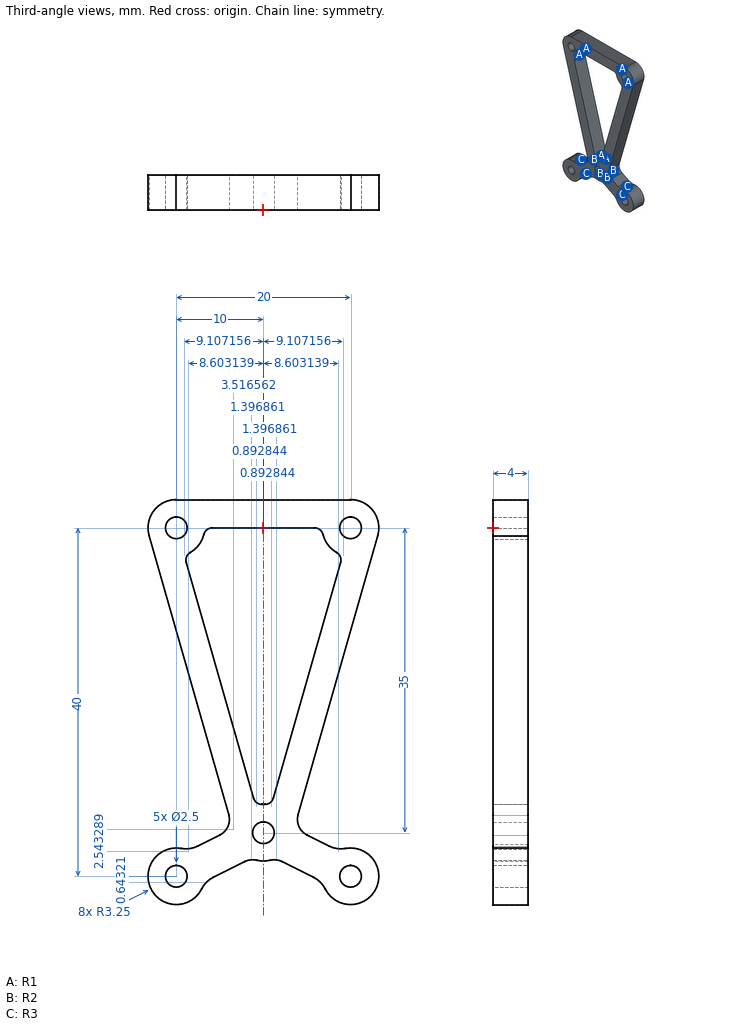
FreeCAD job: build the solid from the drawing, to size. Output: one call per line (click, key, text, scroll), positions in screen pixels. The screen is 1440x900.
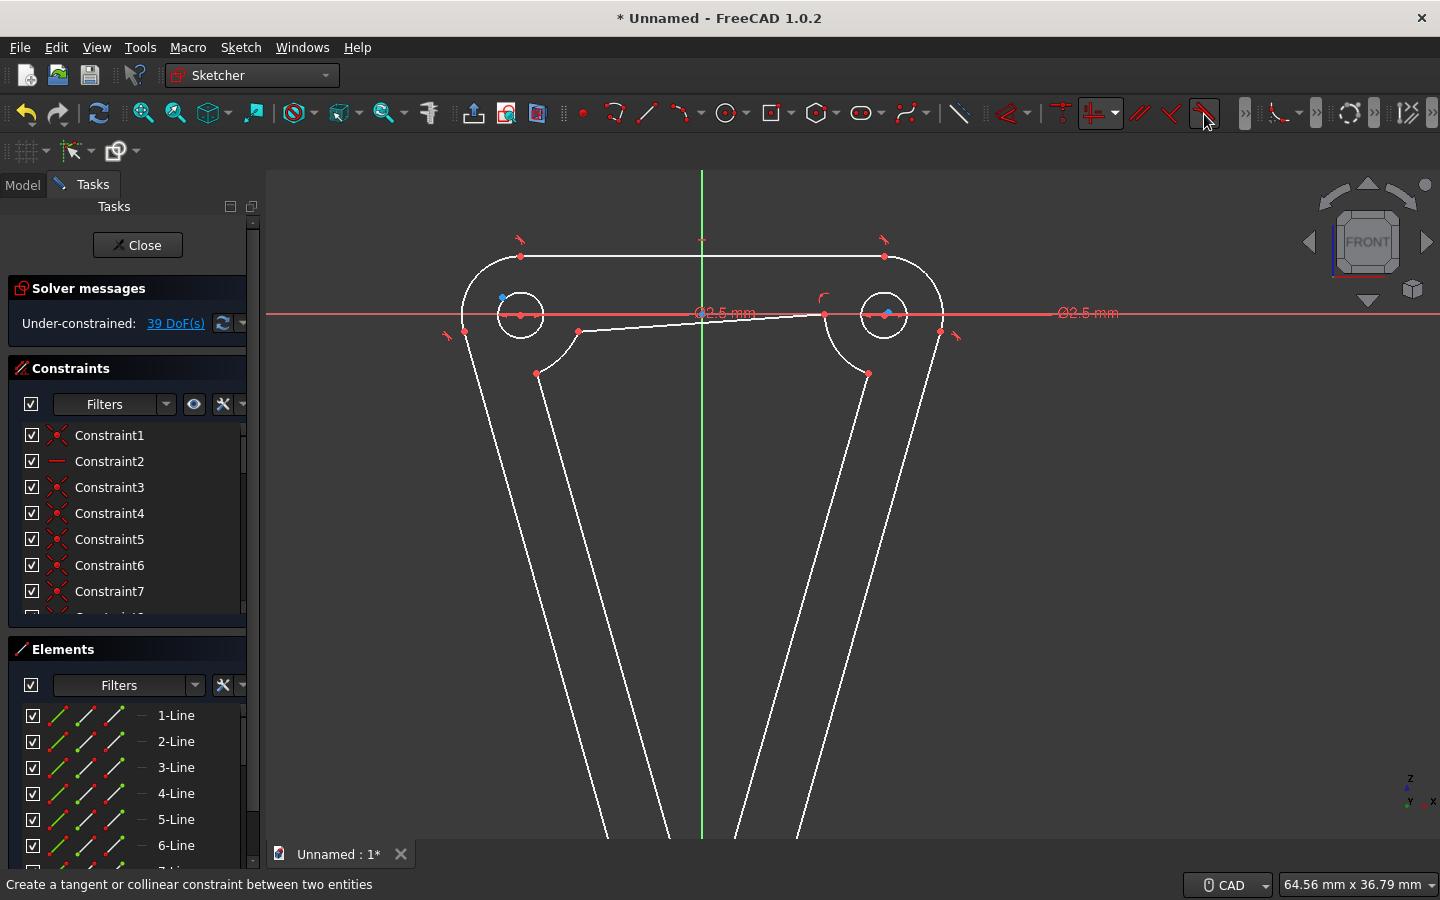
click(653, 327)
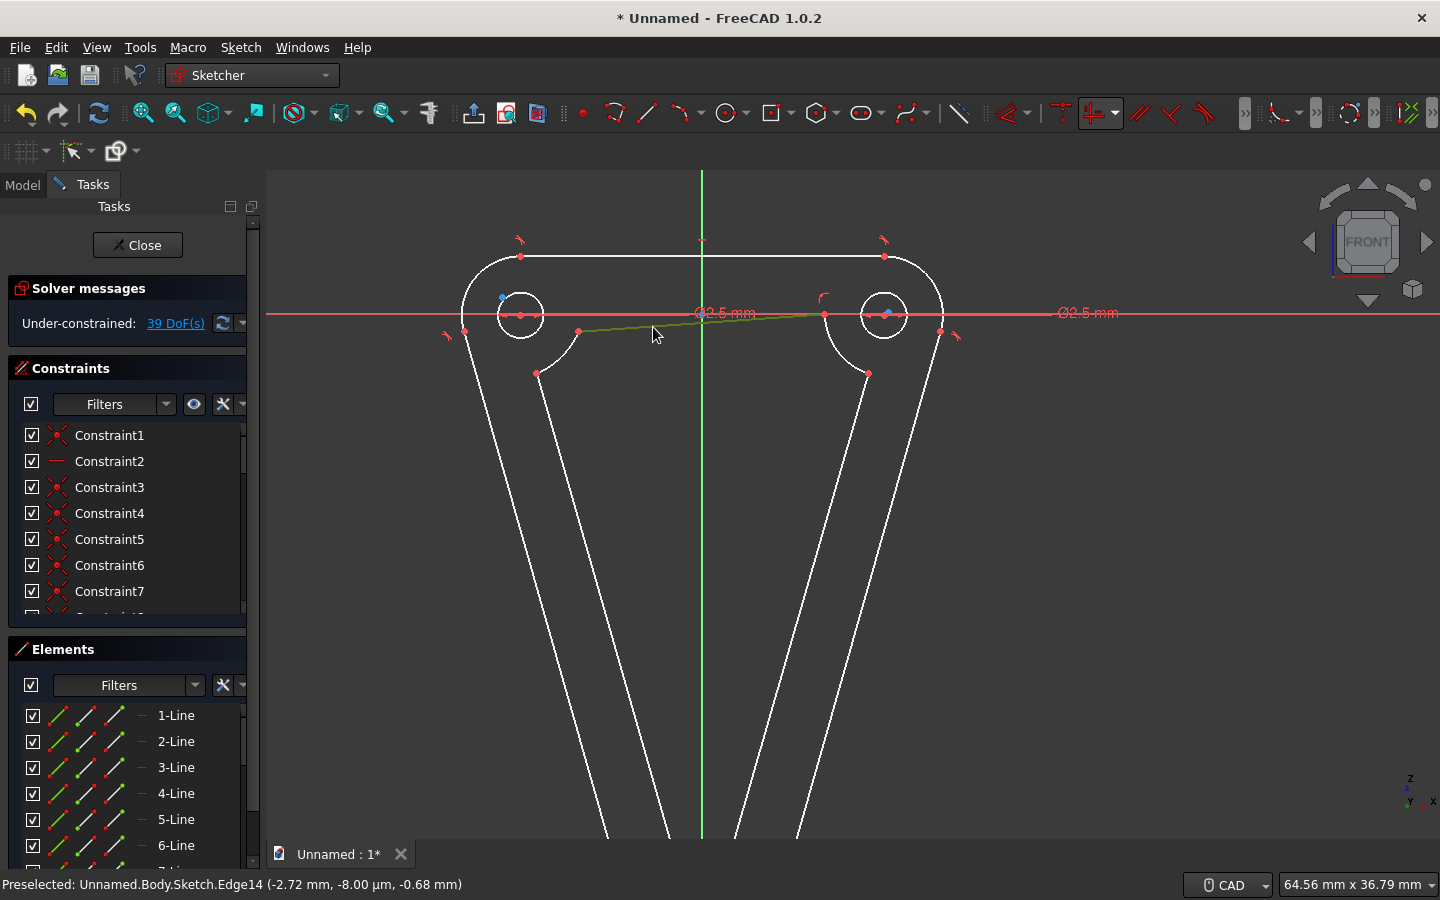
key(h)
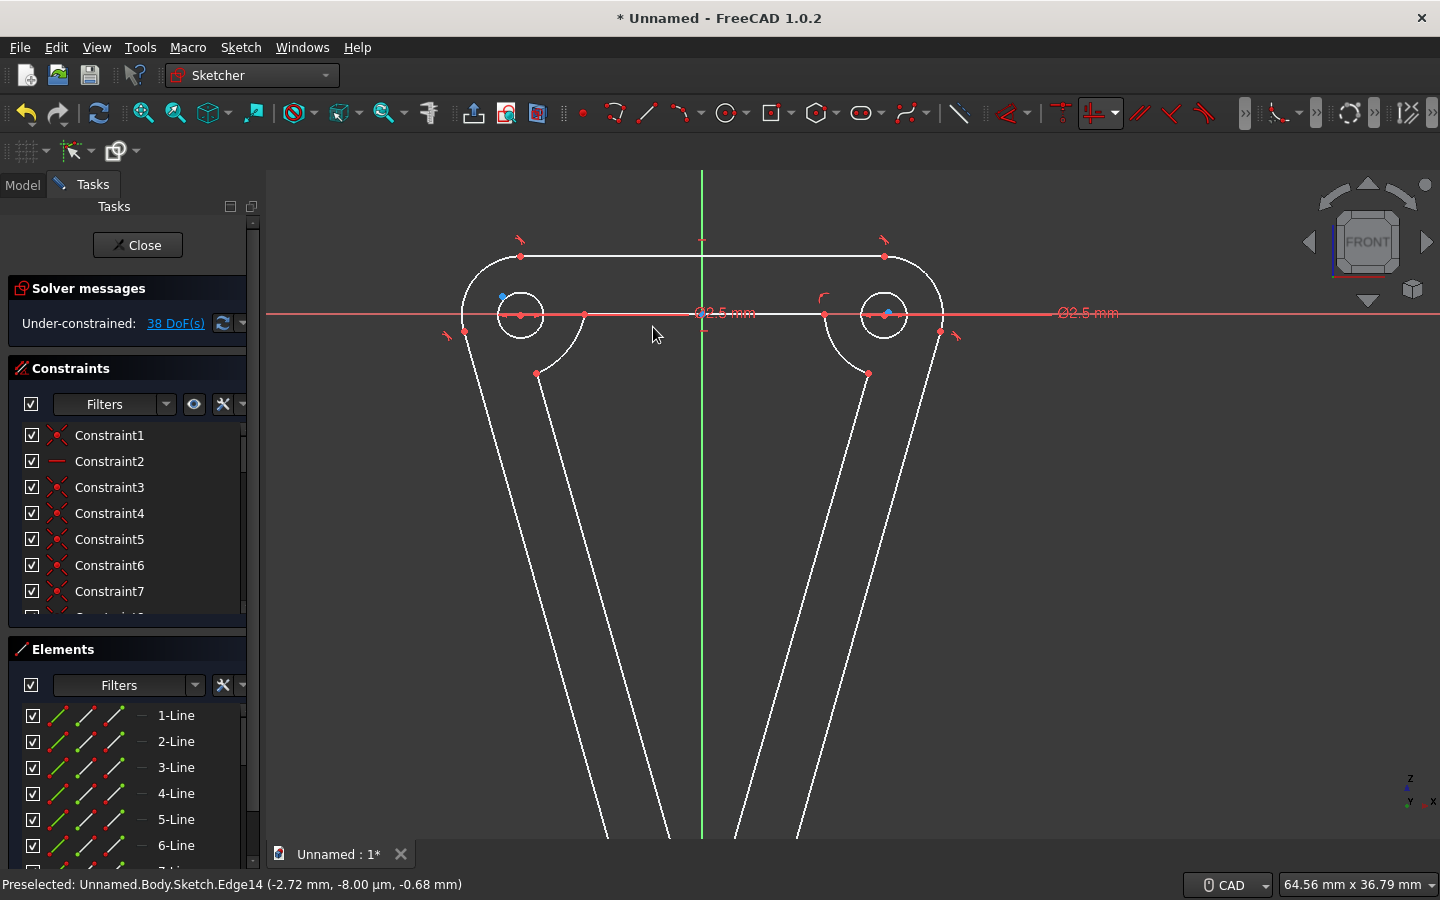
scroll(884, 313, down, 3)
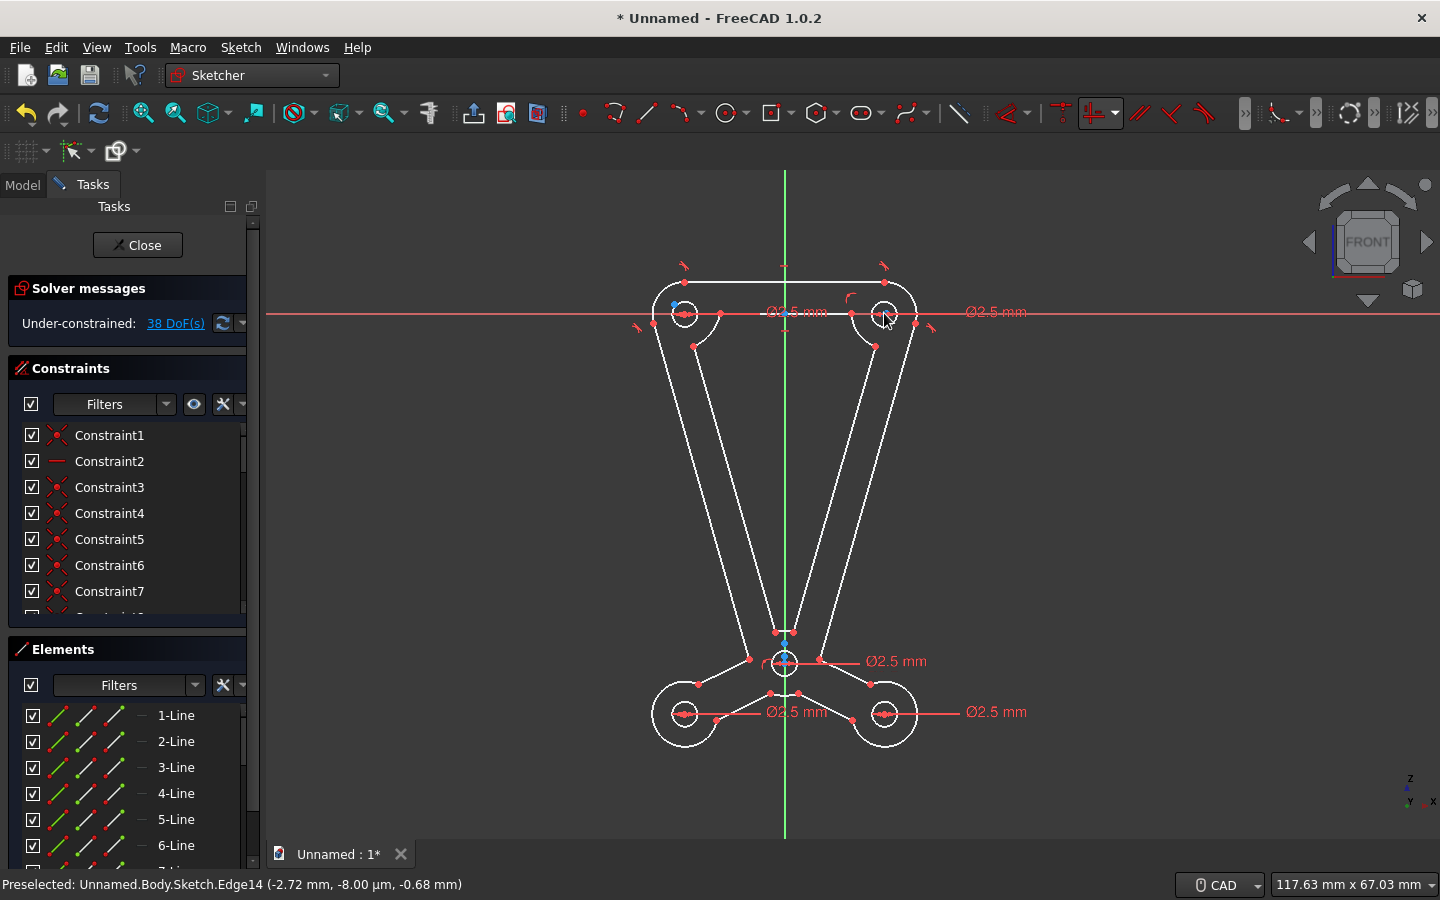
scroll(793, 655, up, 3)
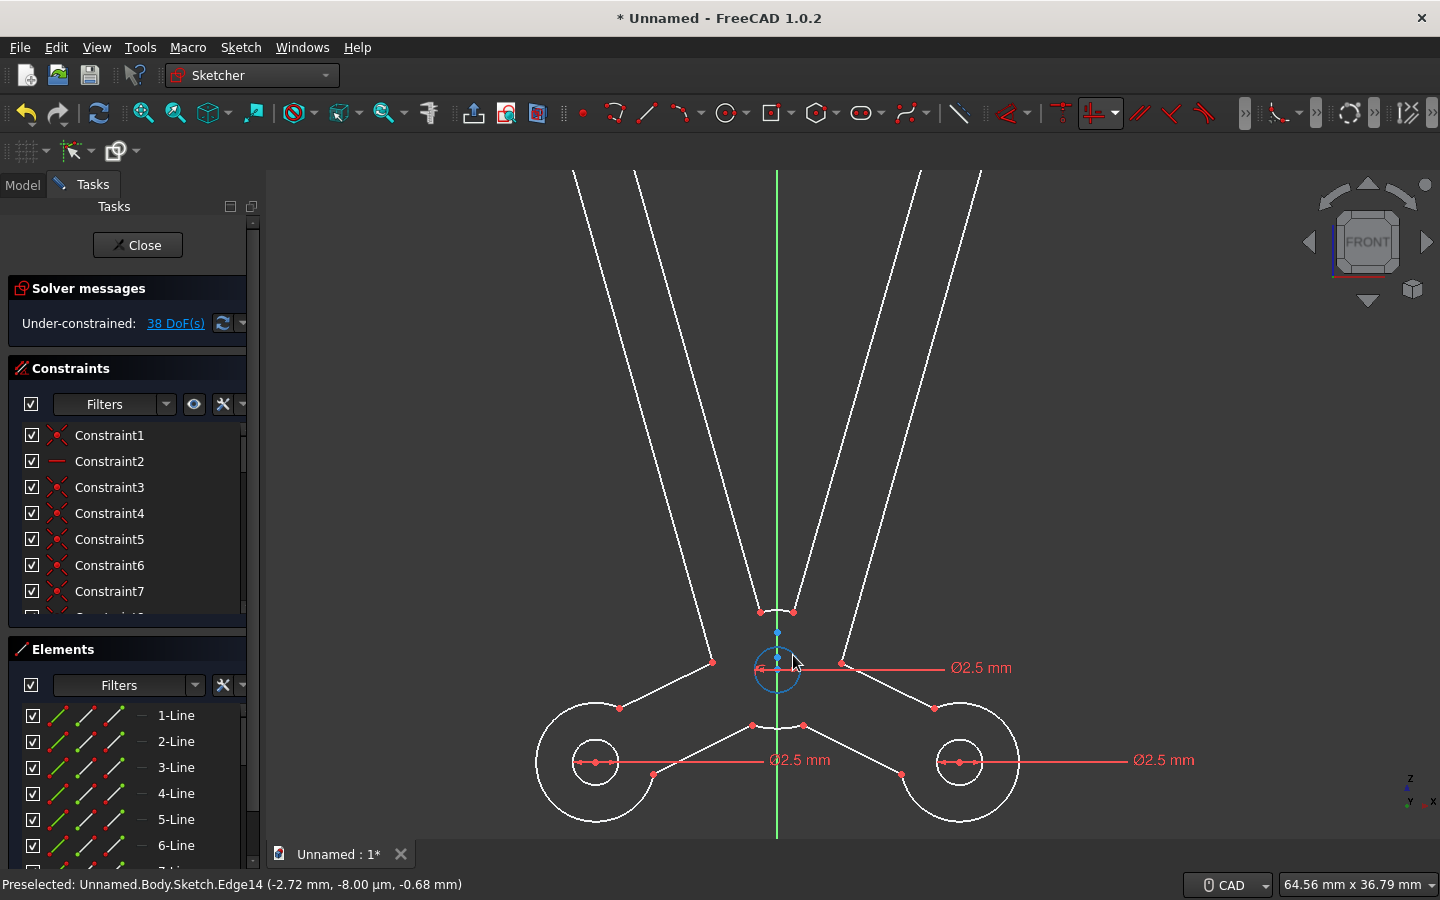
click(793, 654)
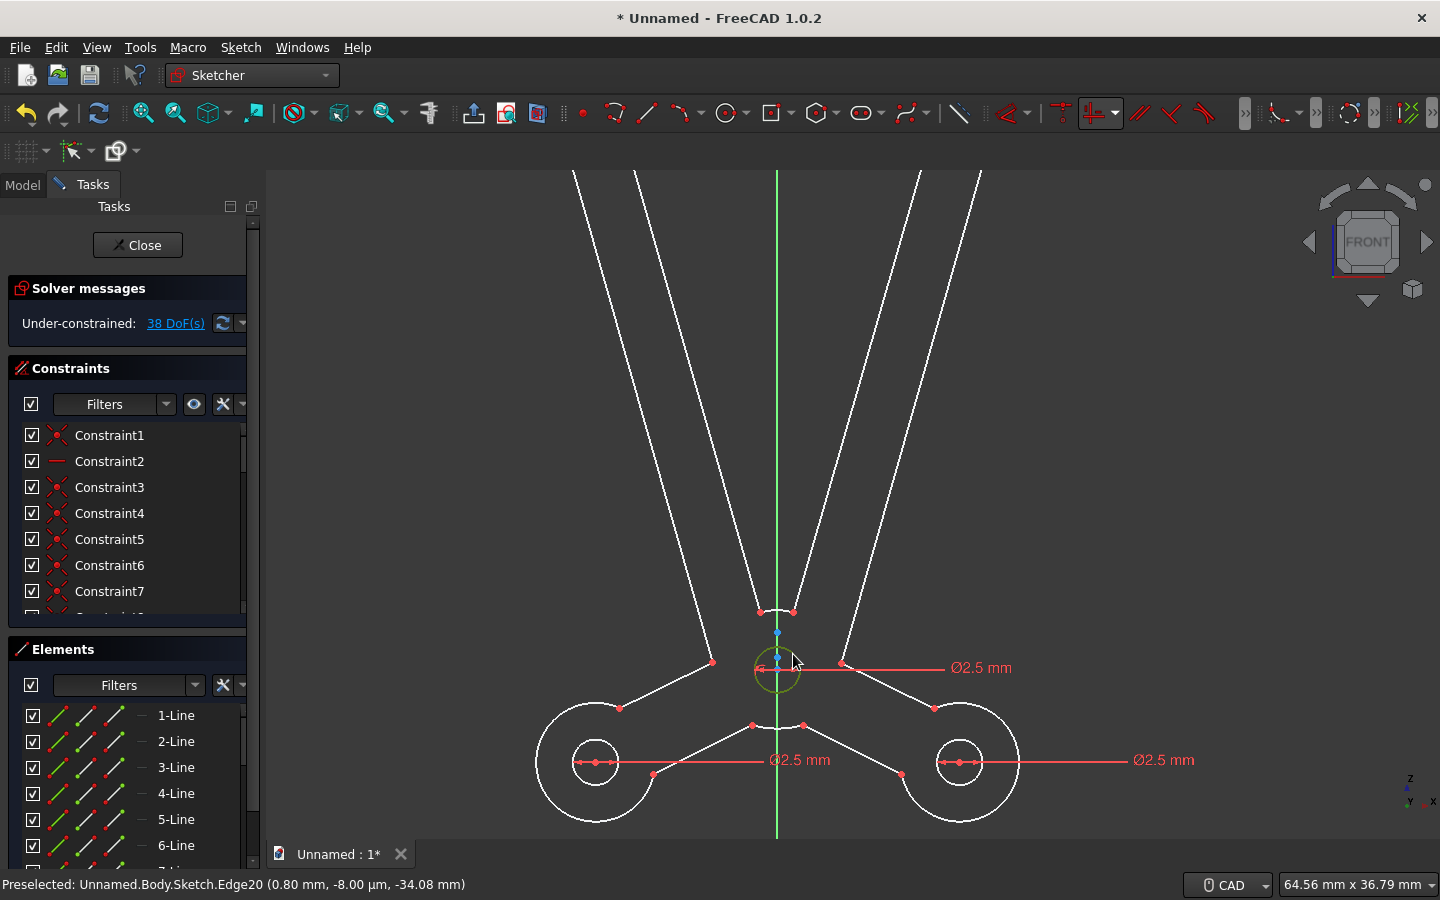
scroll(767, 728, up, 2)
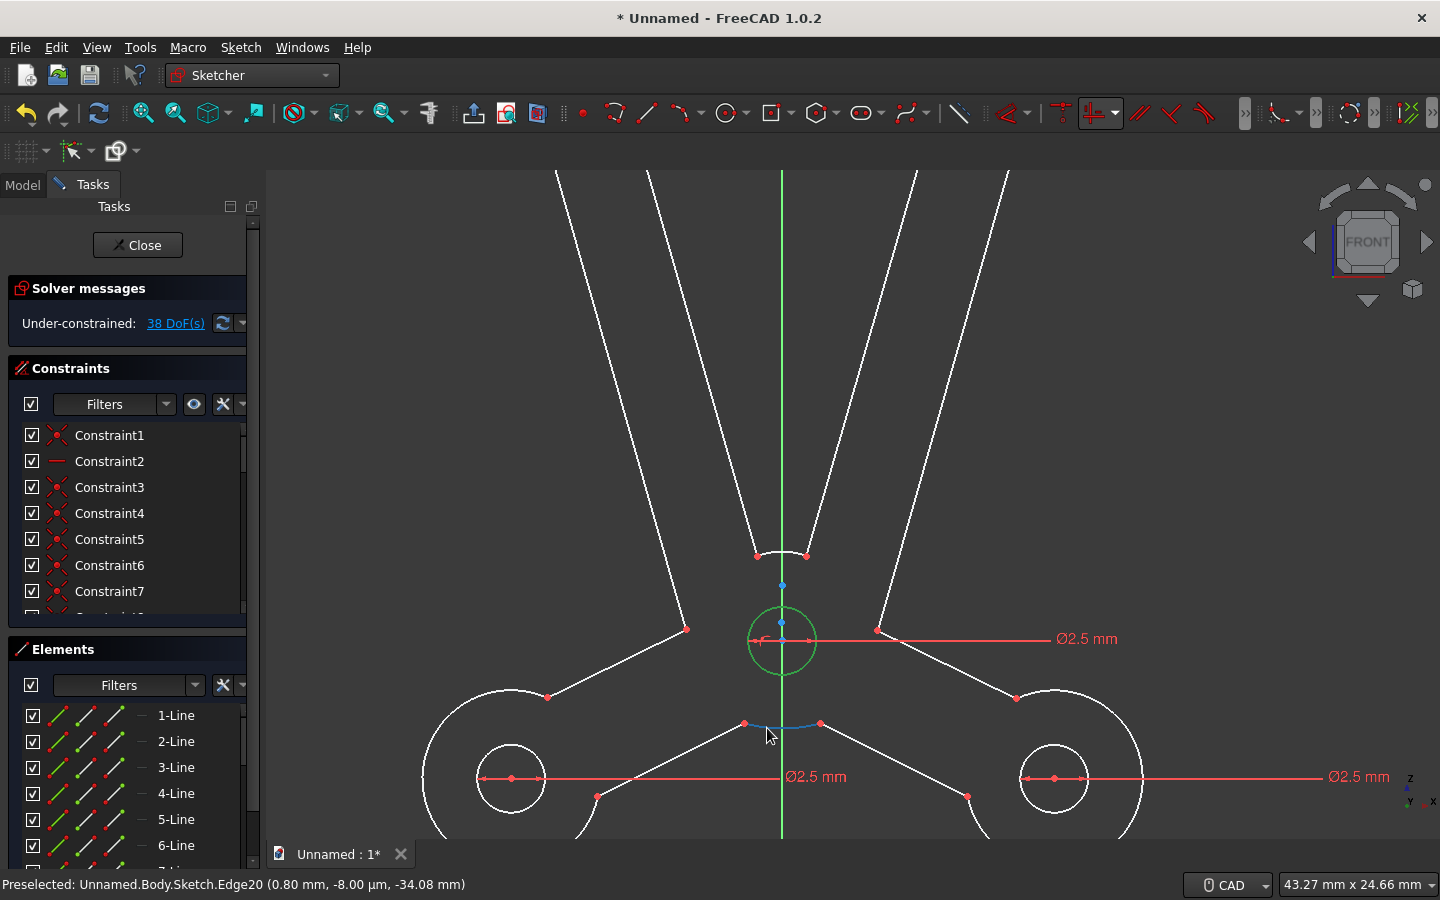
click(767, 728)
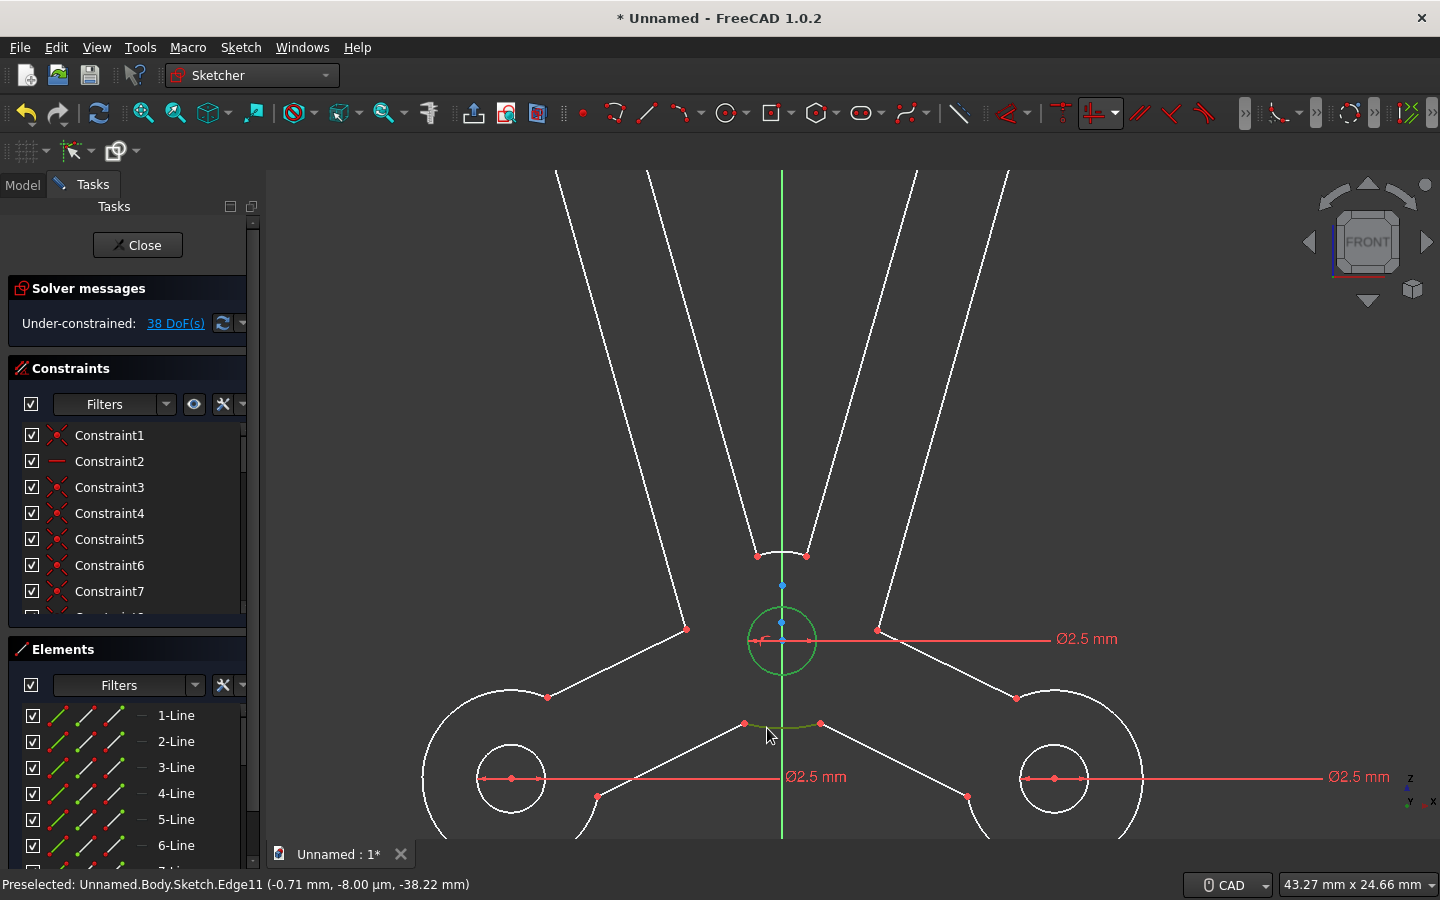
click(1062, 114)